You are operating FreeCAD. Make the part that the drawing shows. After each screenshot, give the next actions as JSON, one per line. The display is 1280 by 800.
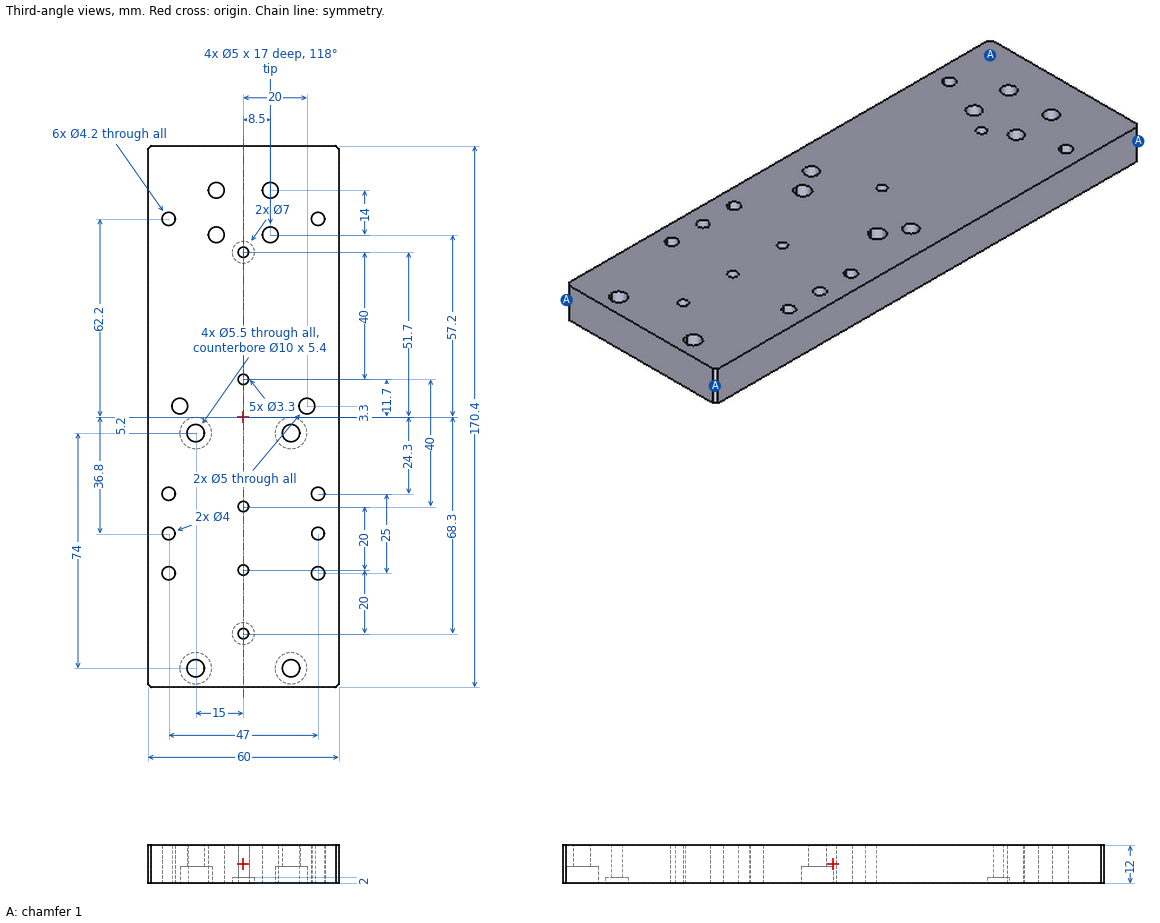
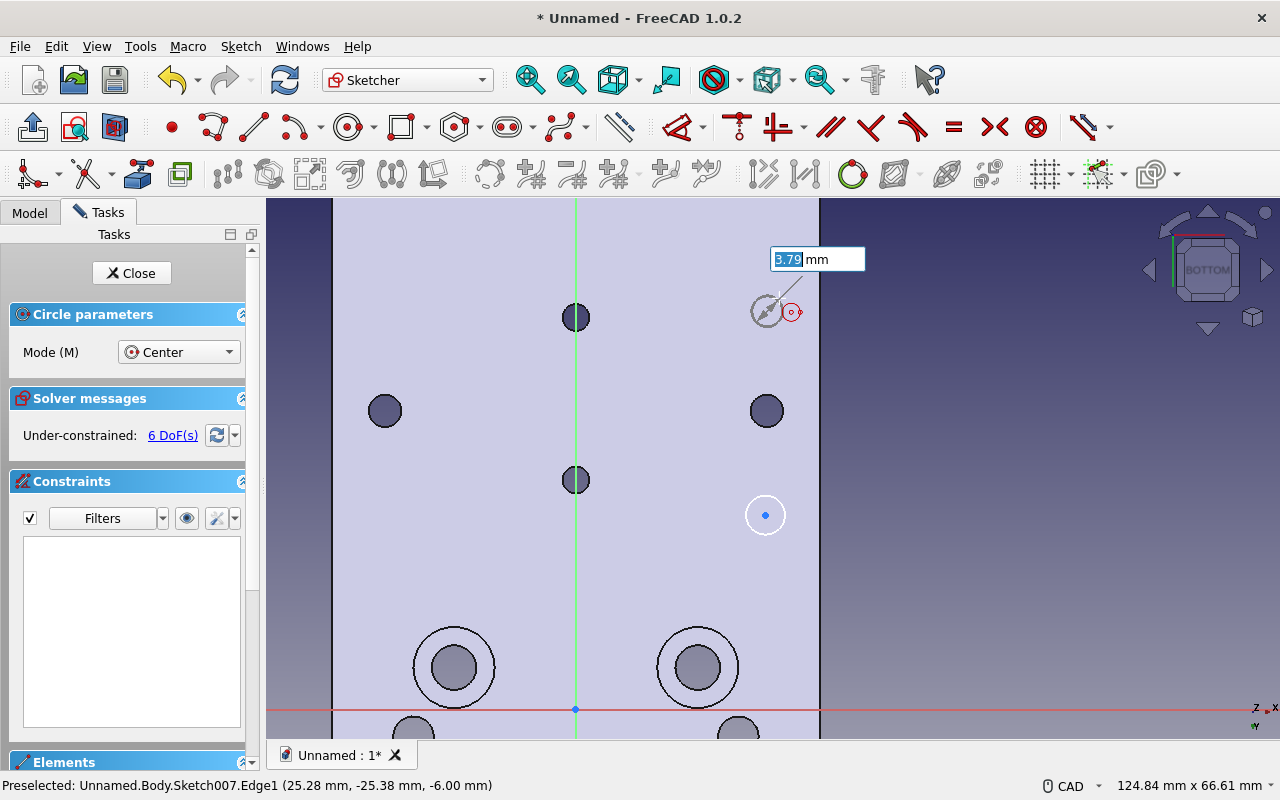
{"action": "left_click", "coordinate": [779, 297]}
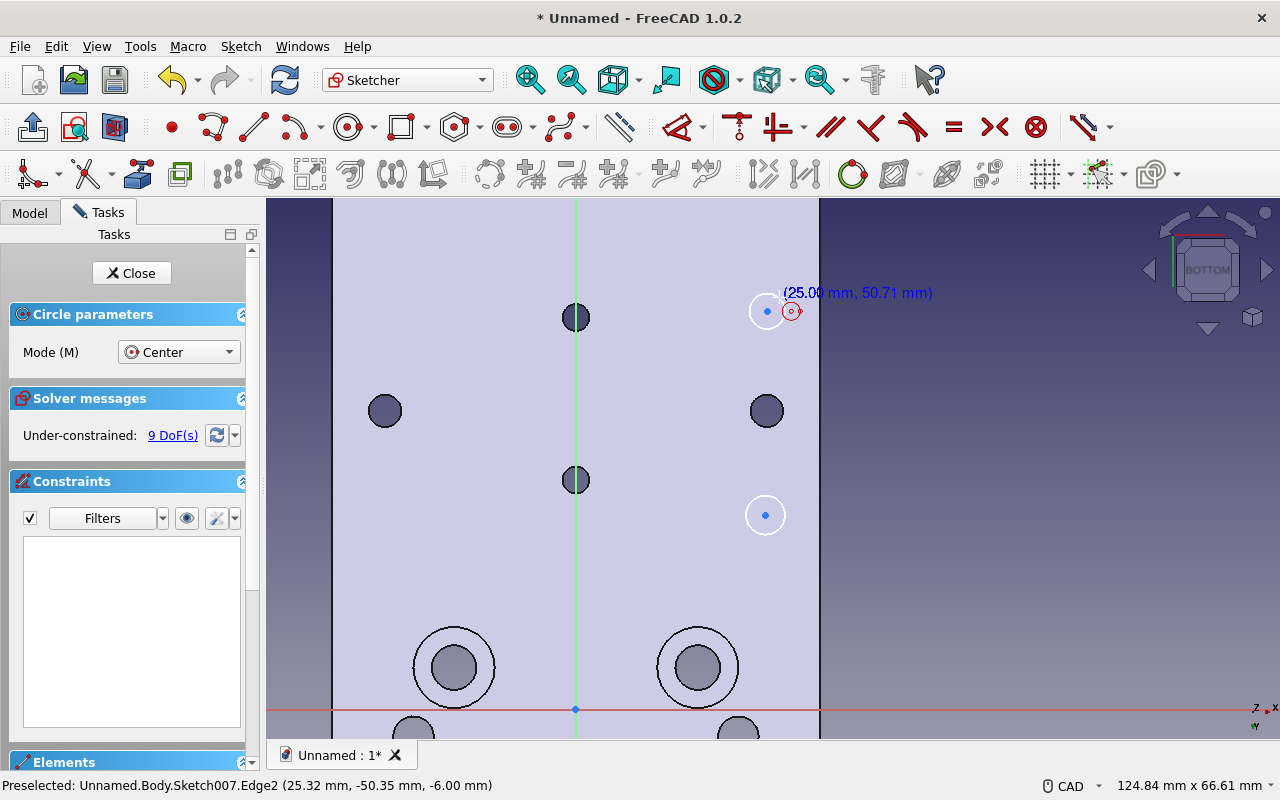
{"action": "scroll", "coordinate": [385, 309], "scroll_direction": "up", "scroll_amount": 2}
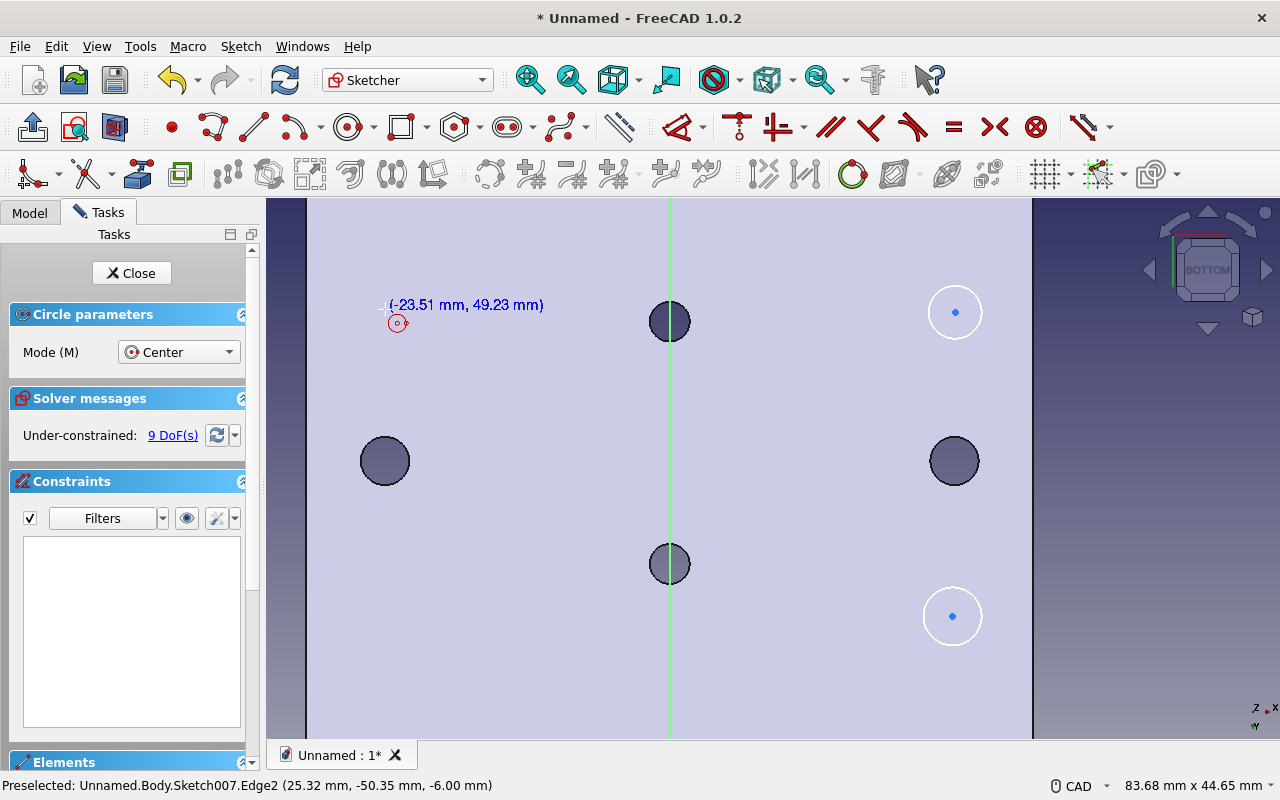
{"action": "scroll", "coordinate": [716, 299], "scroll_direction": "down", "scroll_amount": 7}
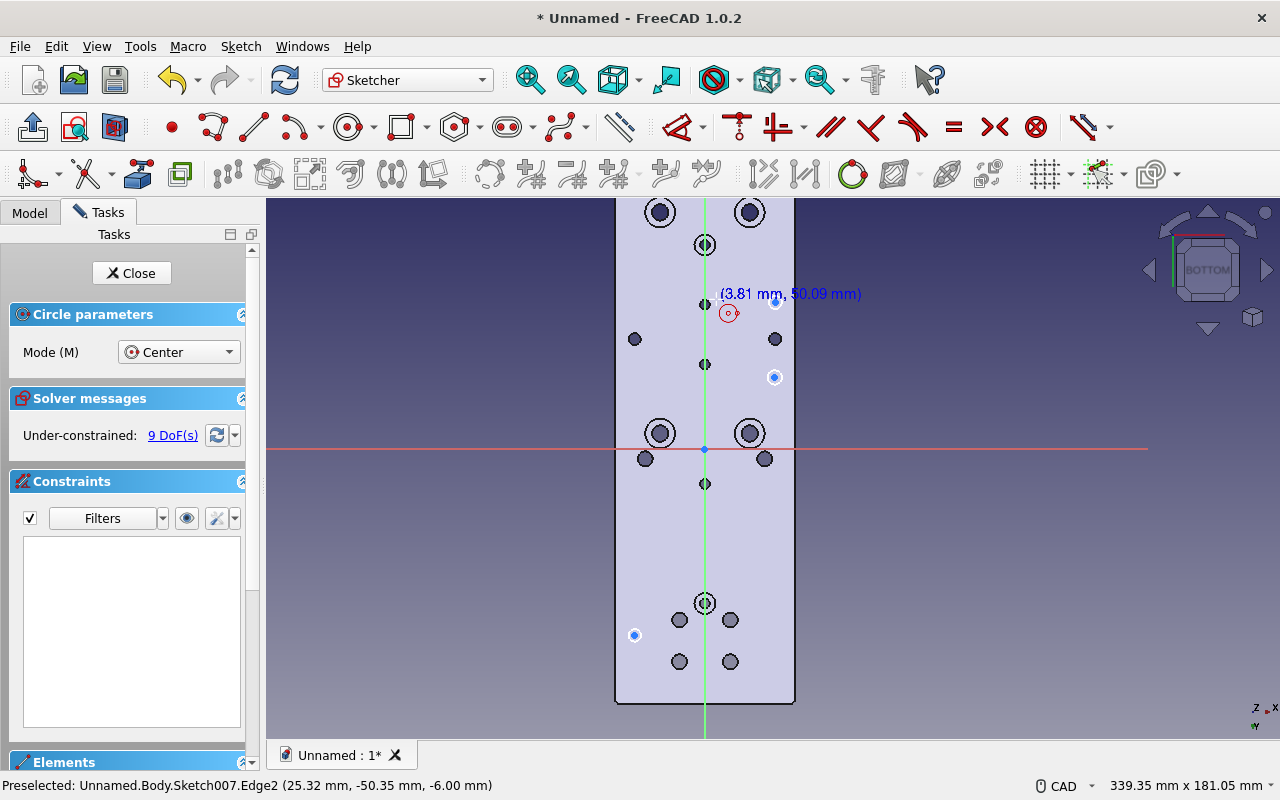
{"action": "left_click", "coordinate": [635, 302]}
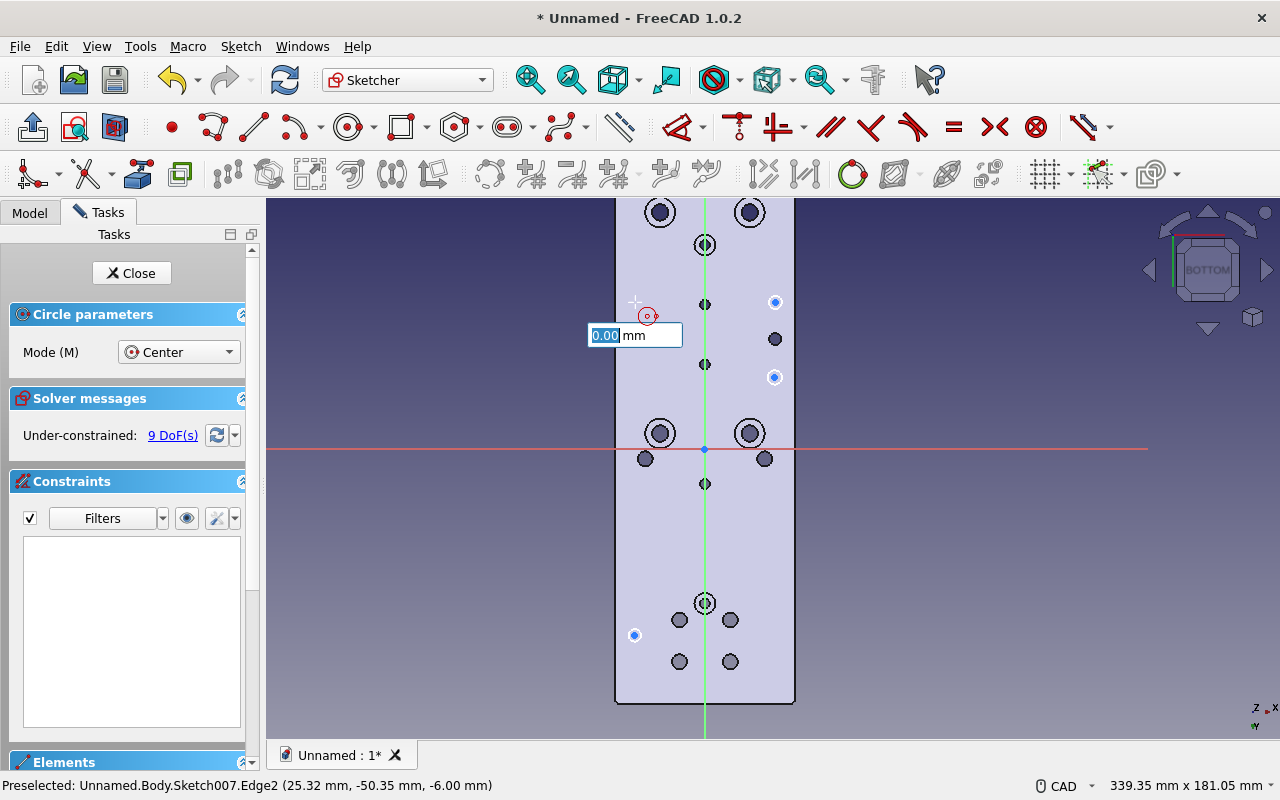
{"action": "scroll", "coordinate": [639, 297], "scroll_direction": "up", "scroll_amount": 5}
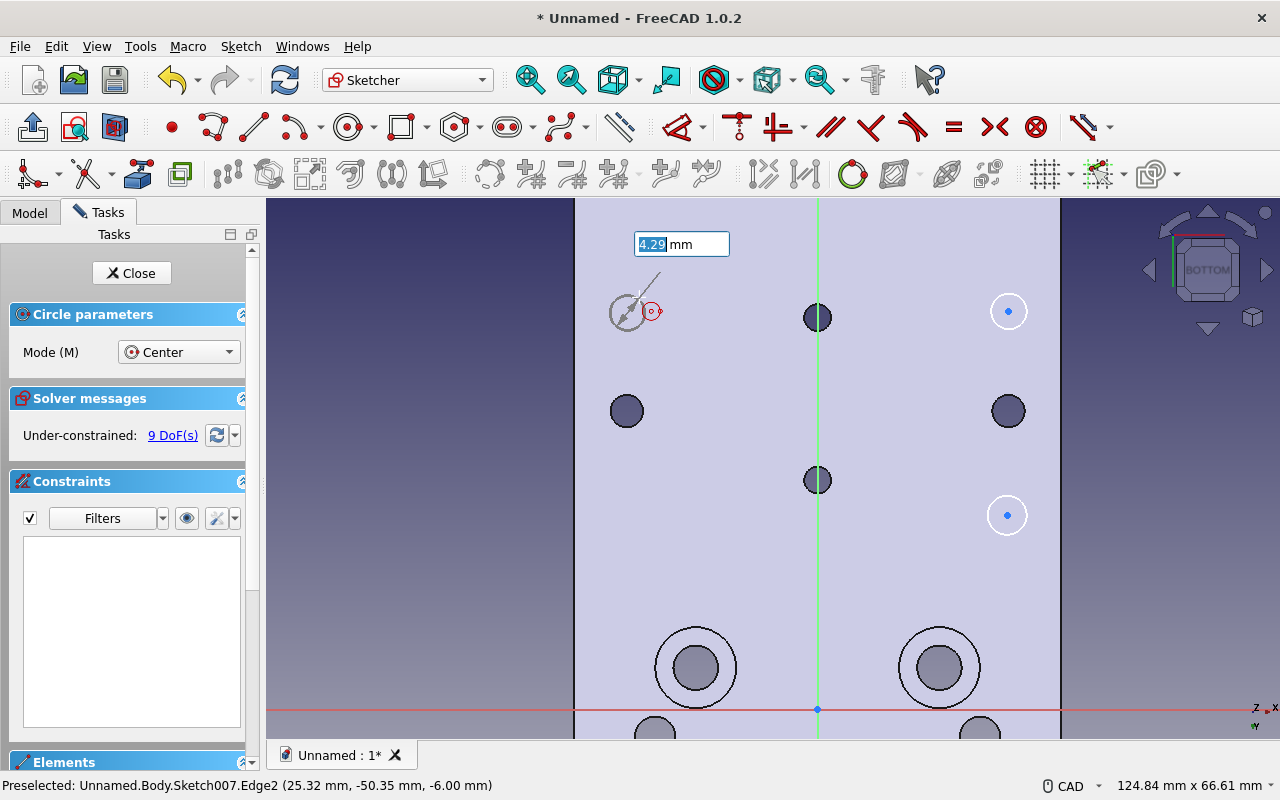
{"action": "left_click", "coordinate": [639, 297]}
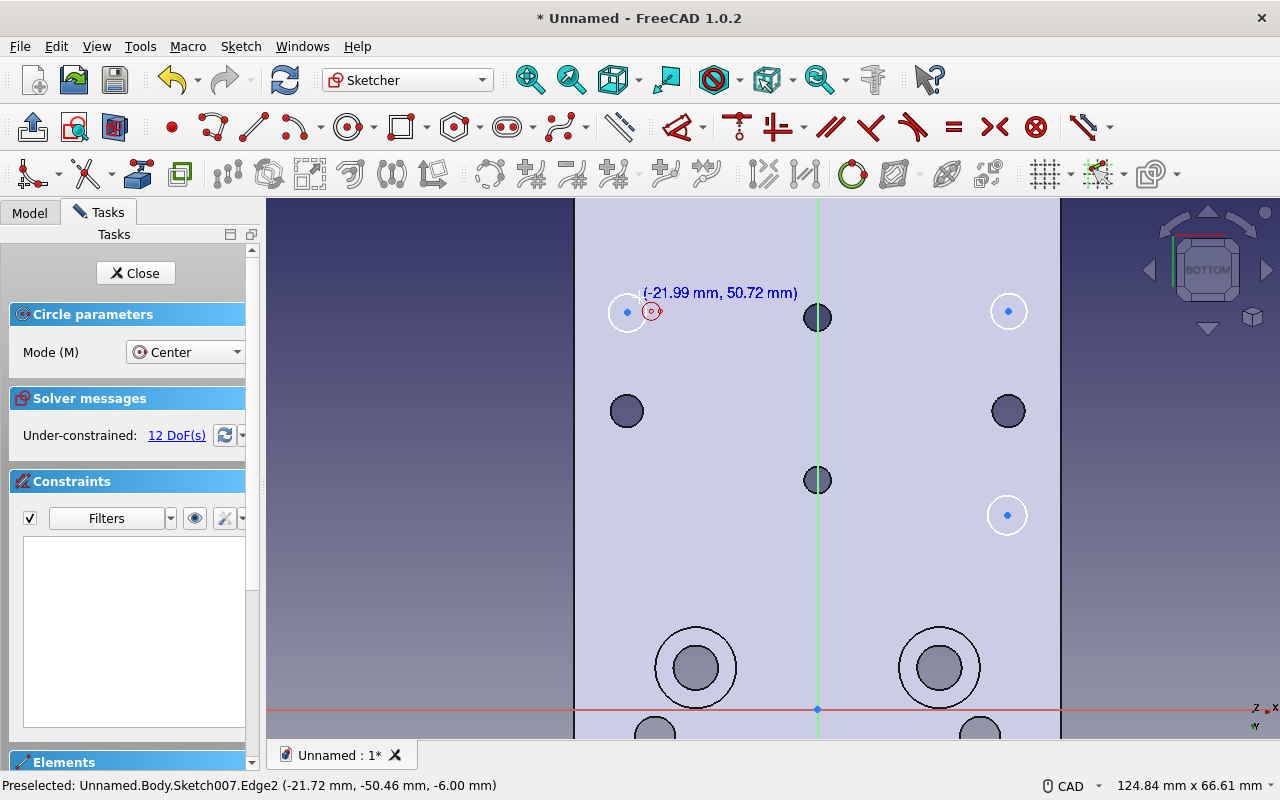
{"action": "scroll", "coordinate": [627, 513], "scroll_direction": "up", "scroll_amount": 2}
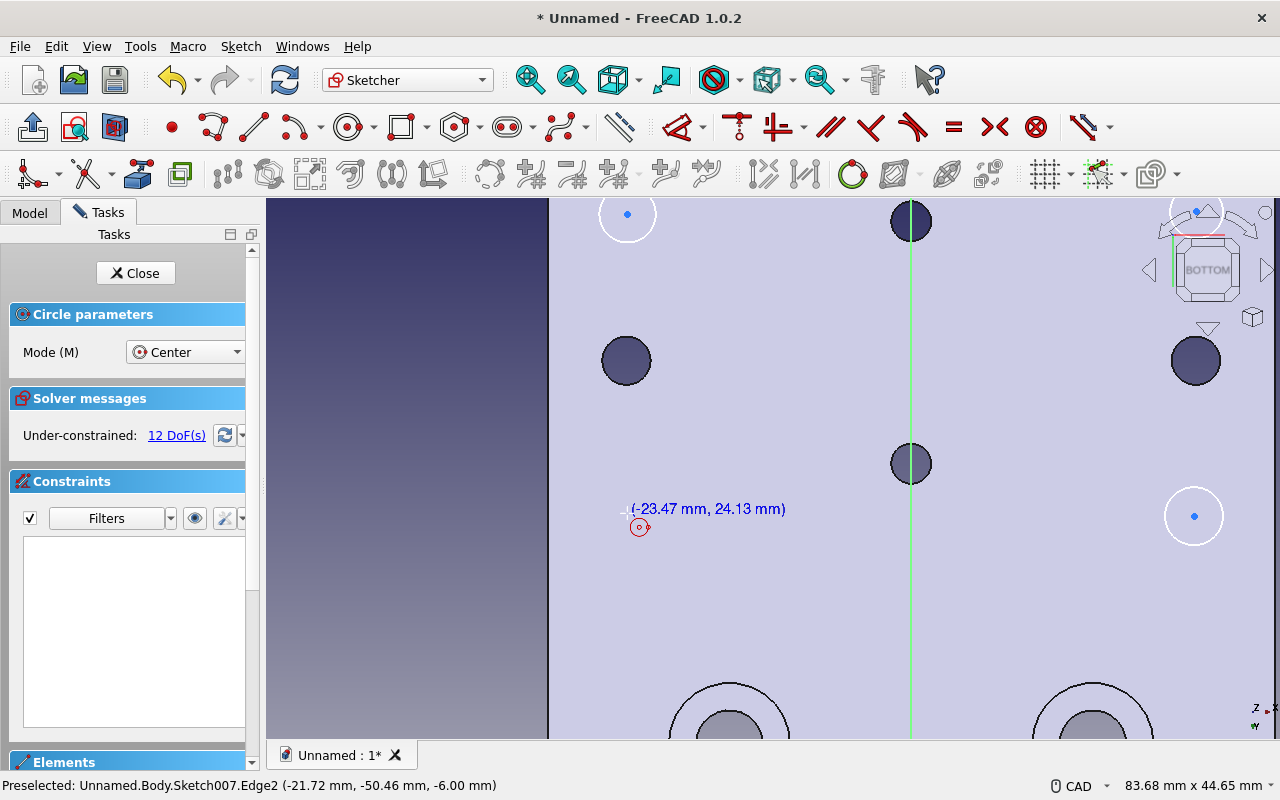
{"action": "scroll", "coordinate": [637, 332], "scroll_direction": "down", "scroll_amount": 7}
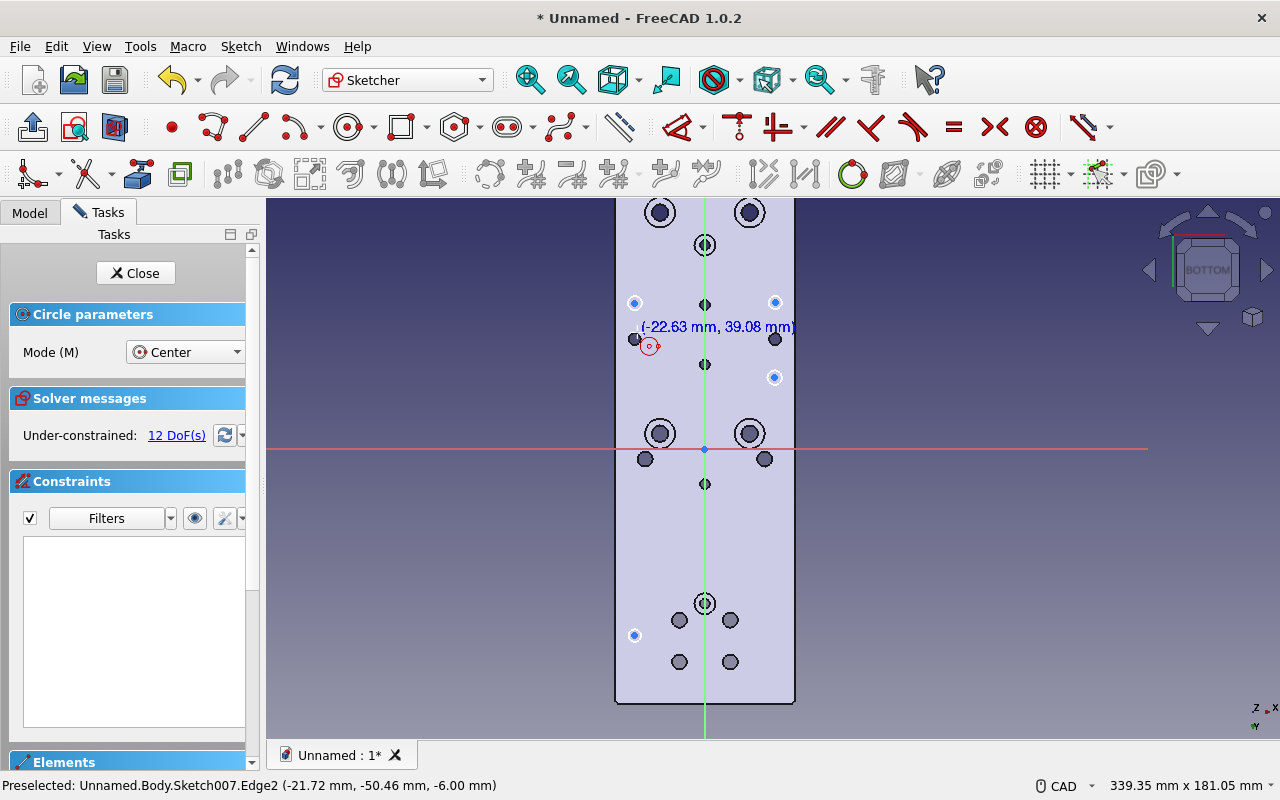
{"action": "left_click", "coordinate": [635, 377]}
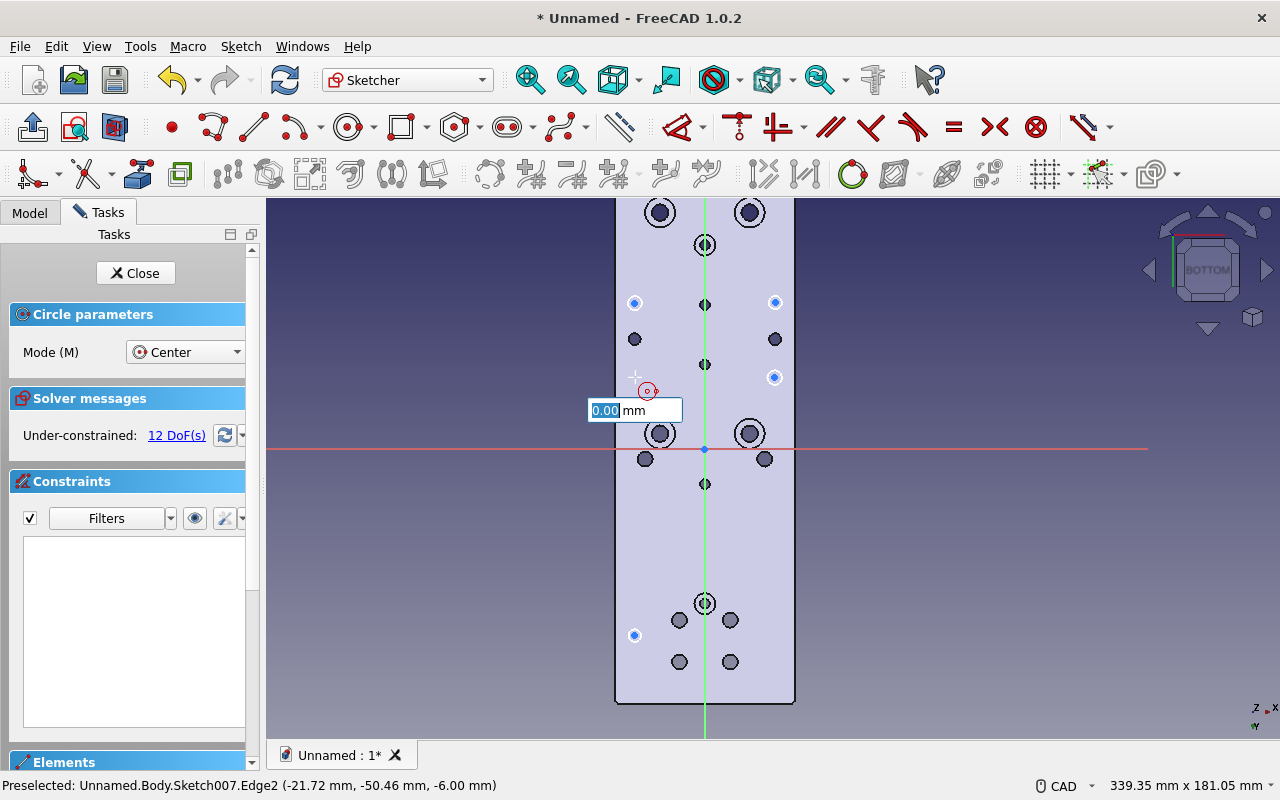
{"action": "scroll", "coordinate": [639, 372], "scroll_direction": "up", "scroll_amount": 5}